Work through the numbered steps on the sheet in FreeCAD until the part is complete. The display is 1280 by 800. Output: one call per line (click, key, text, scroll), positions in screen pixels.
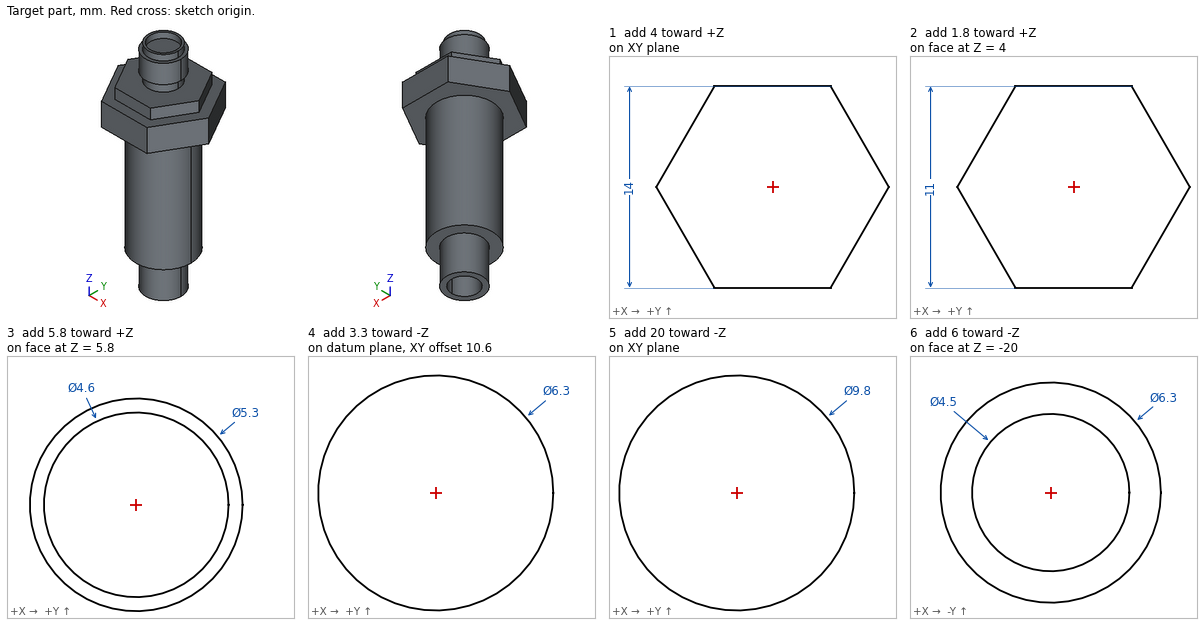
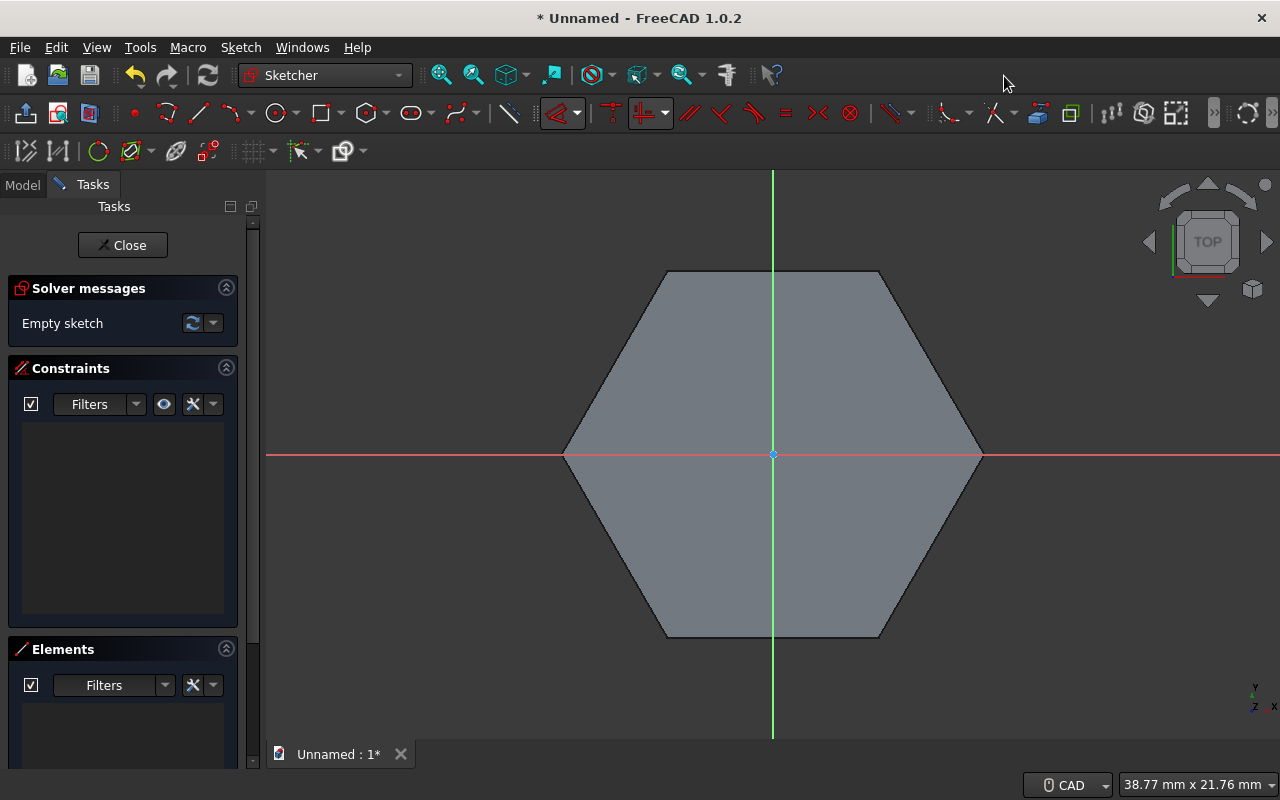
click(366, 114)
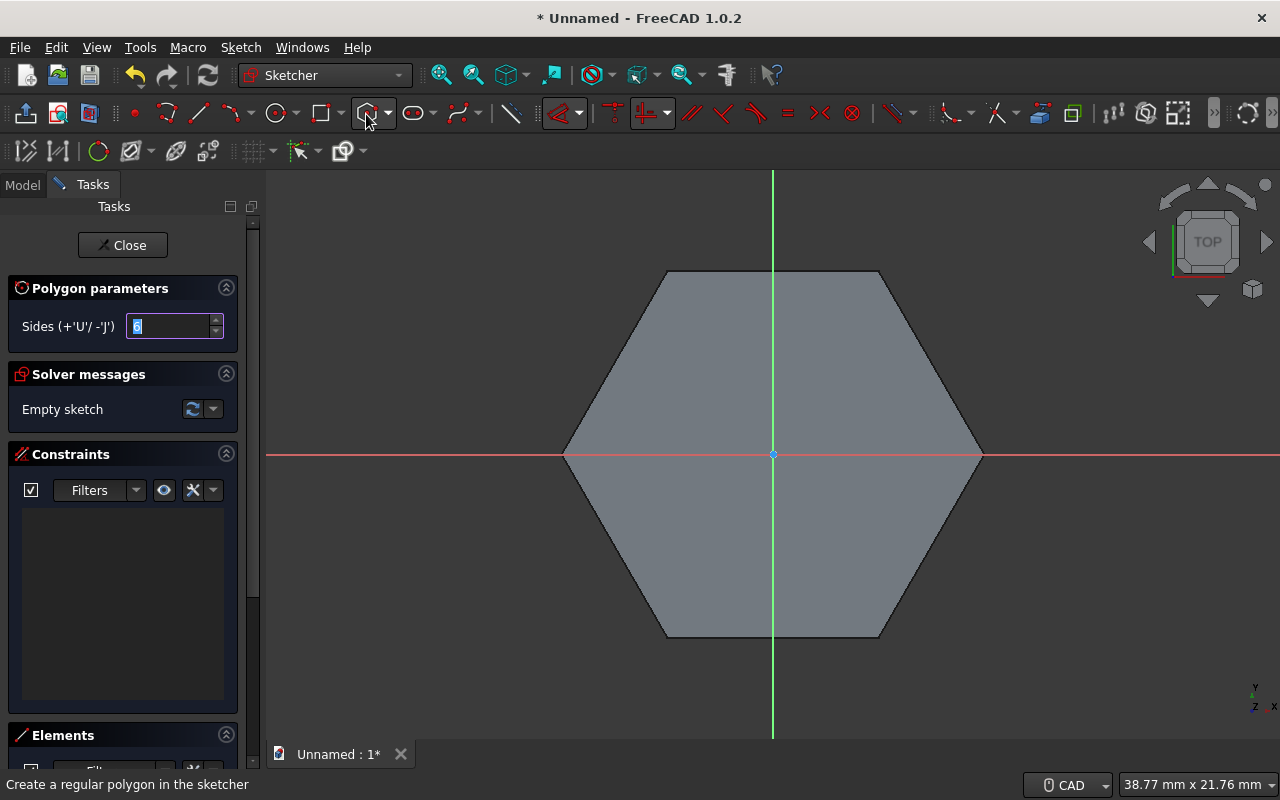
click(773, 454)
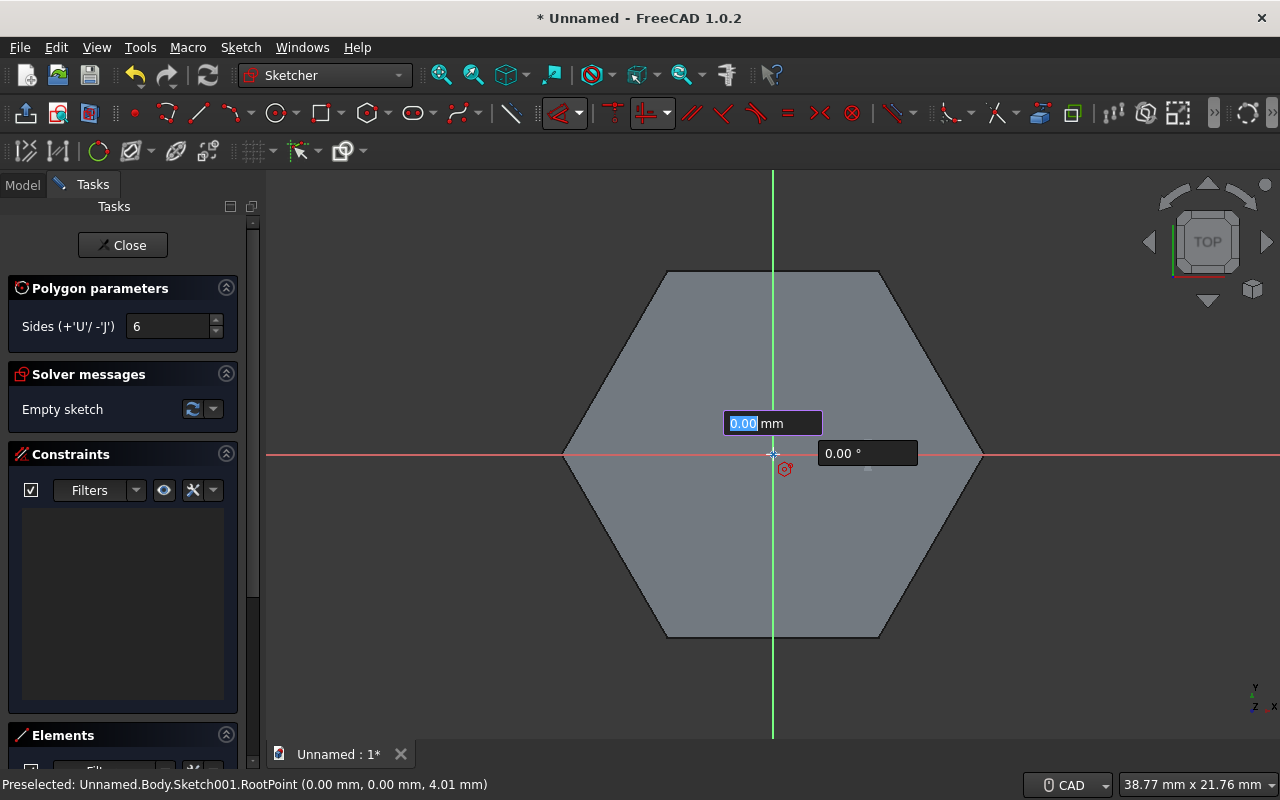
click(939, 454)
right_click(939, 454)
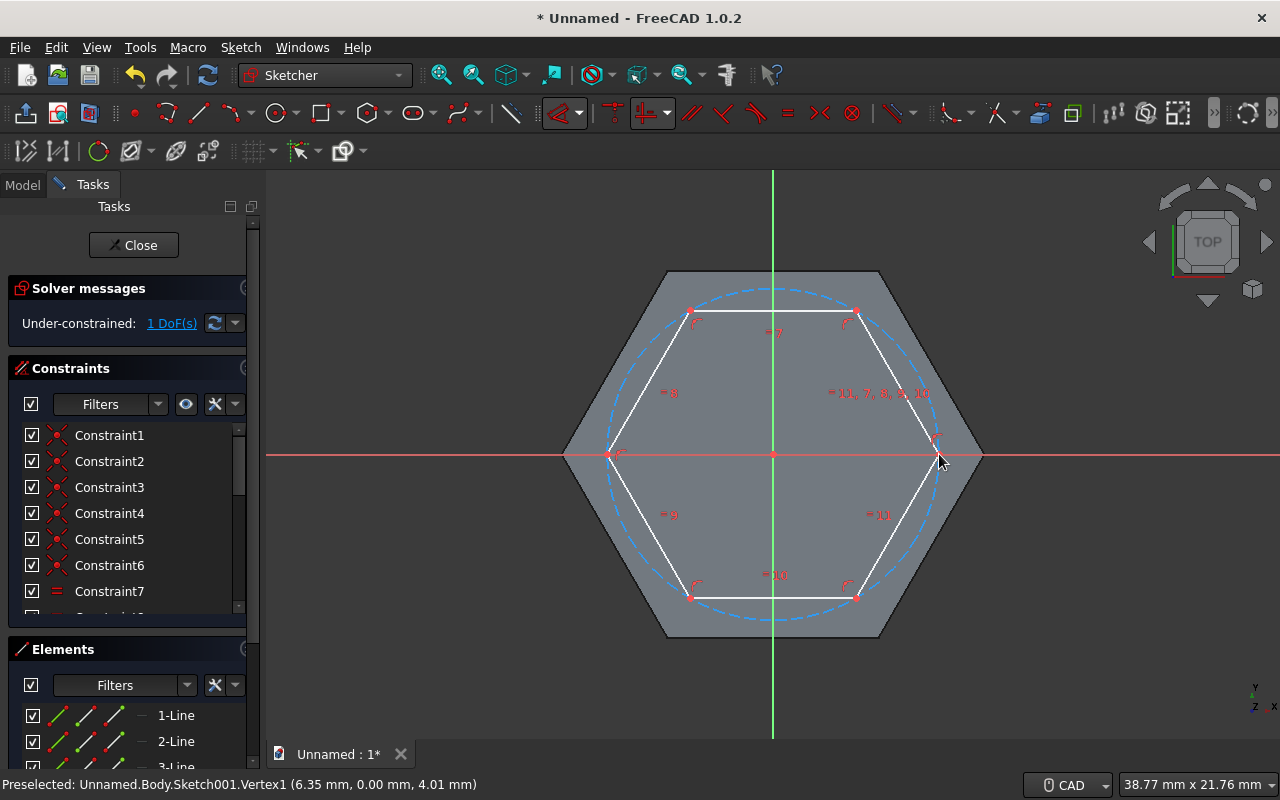
click(690, 598)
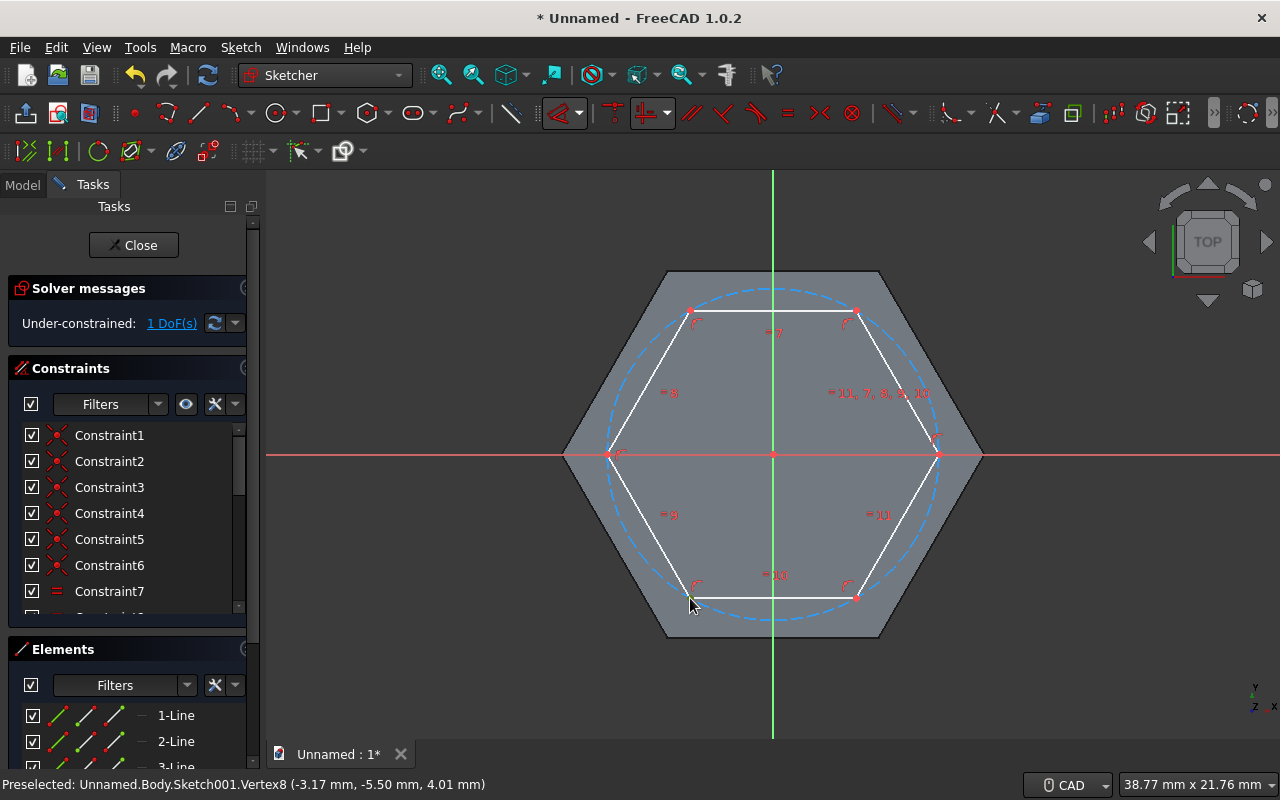
click(856, 311)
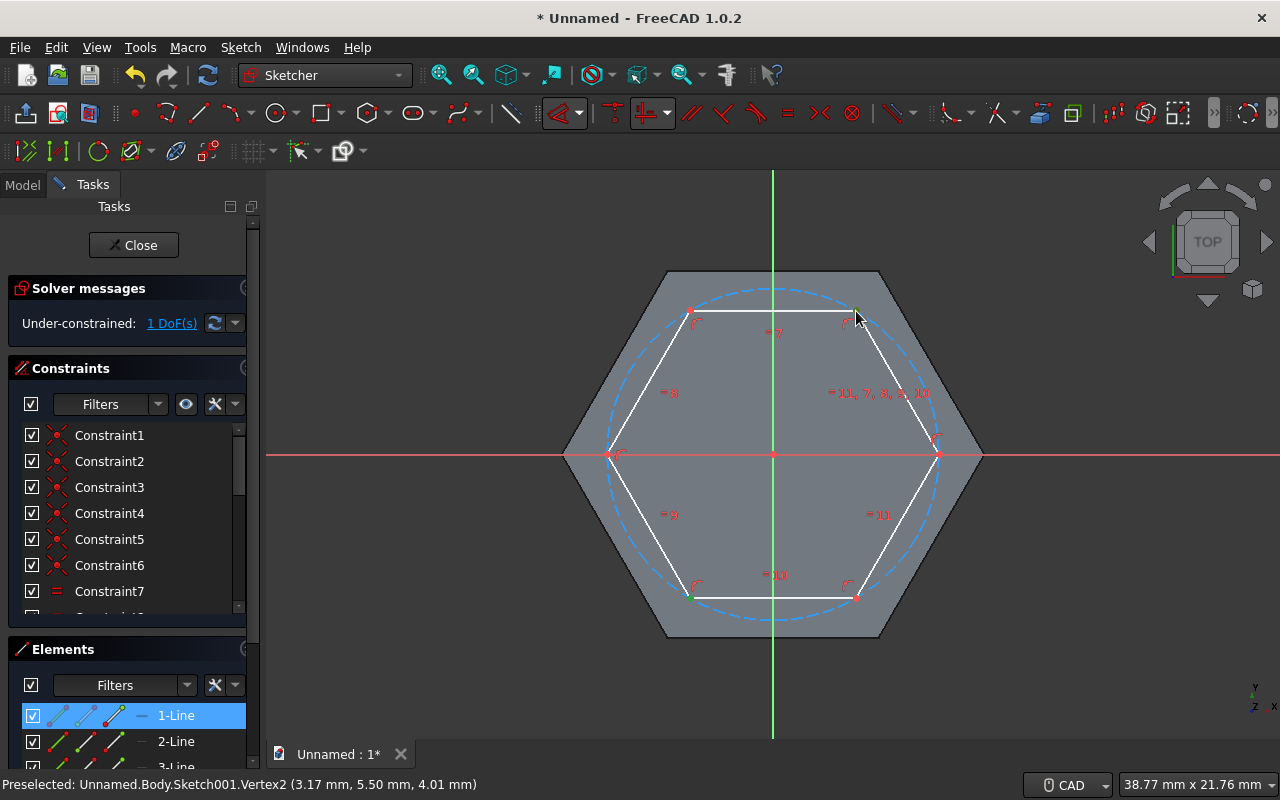
key(i)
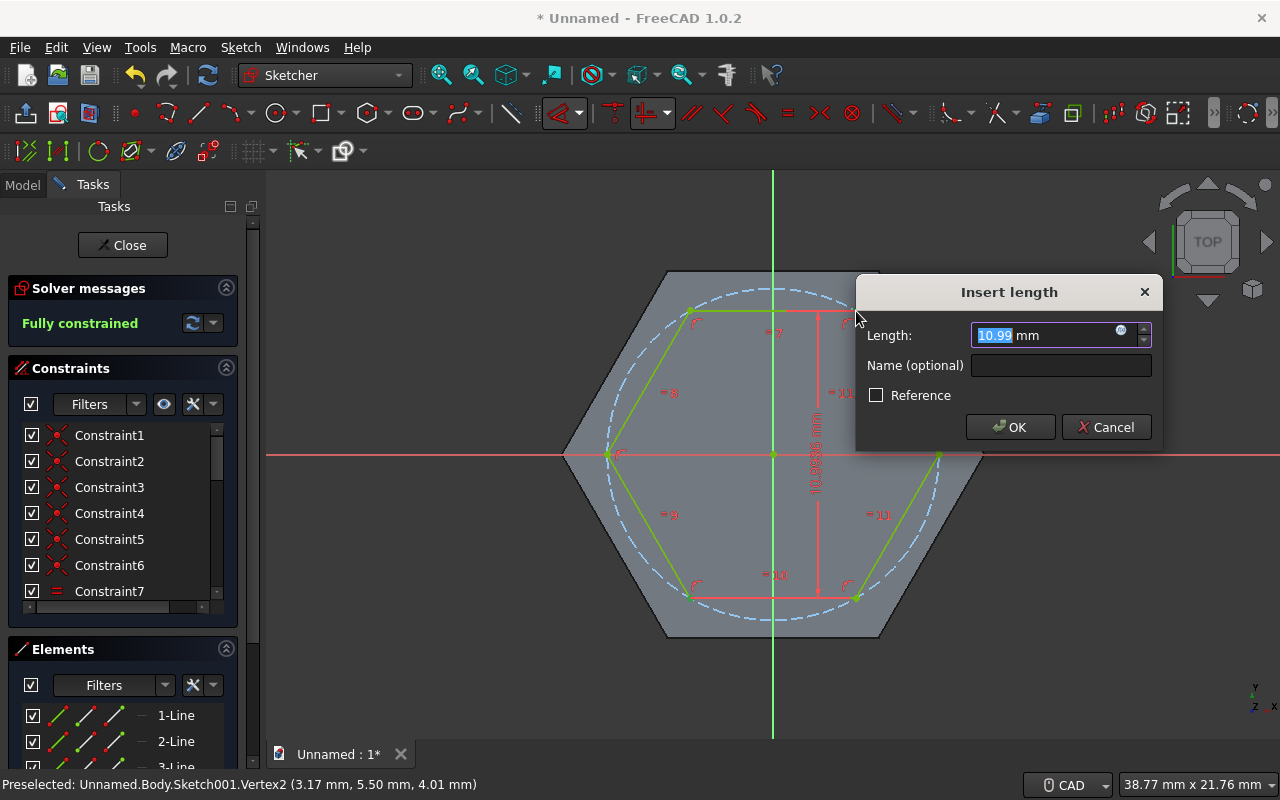
text(11)
key(Return)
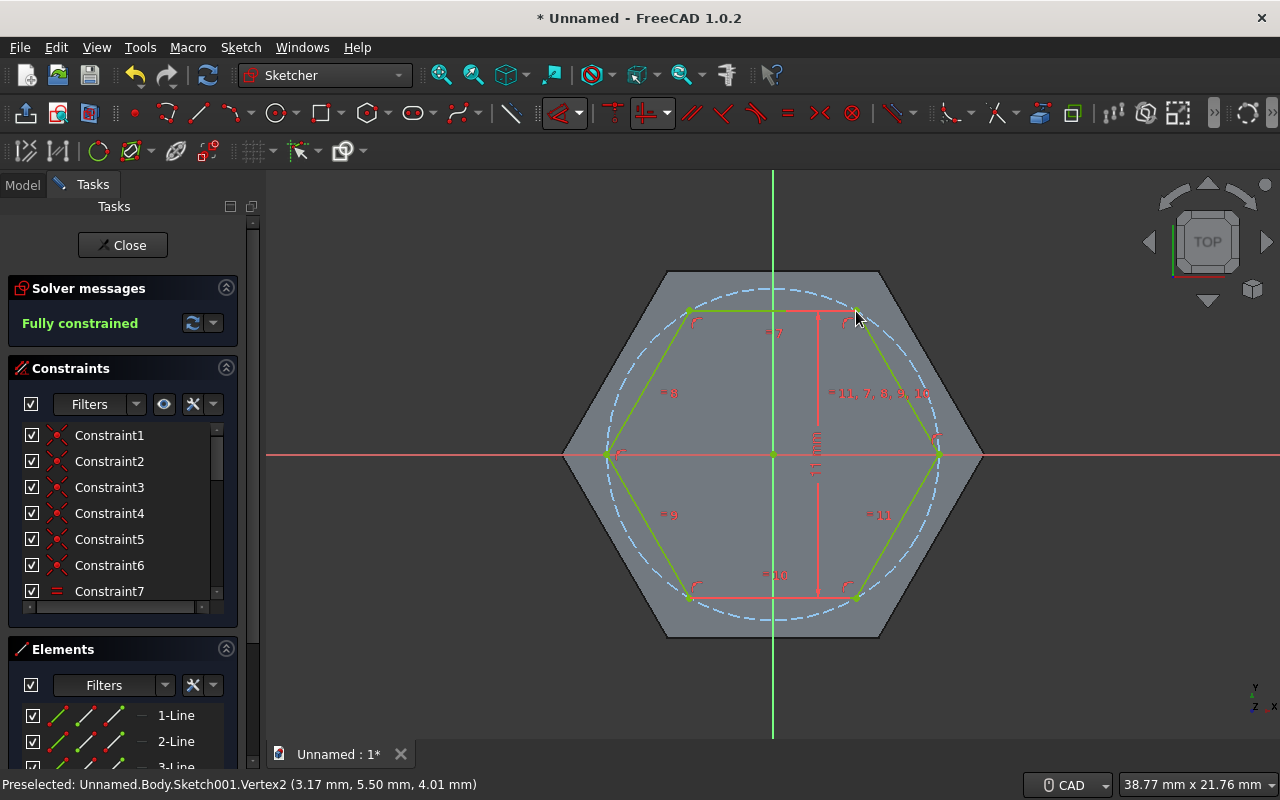
click(123, 245)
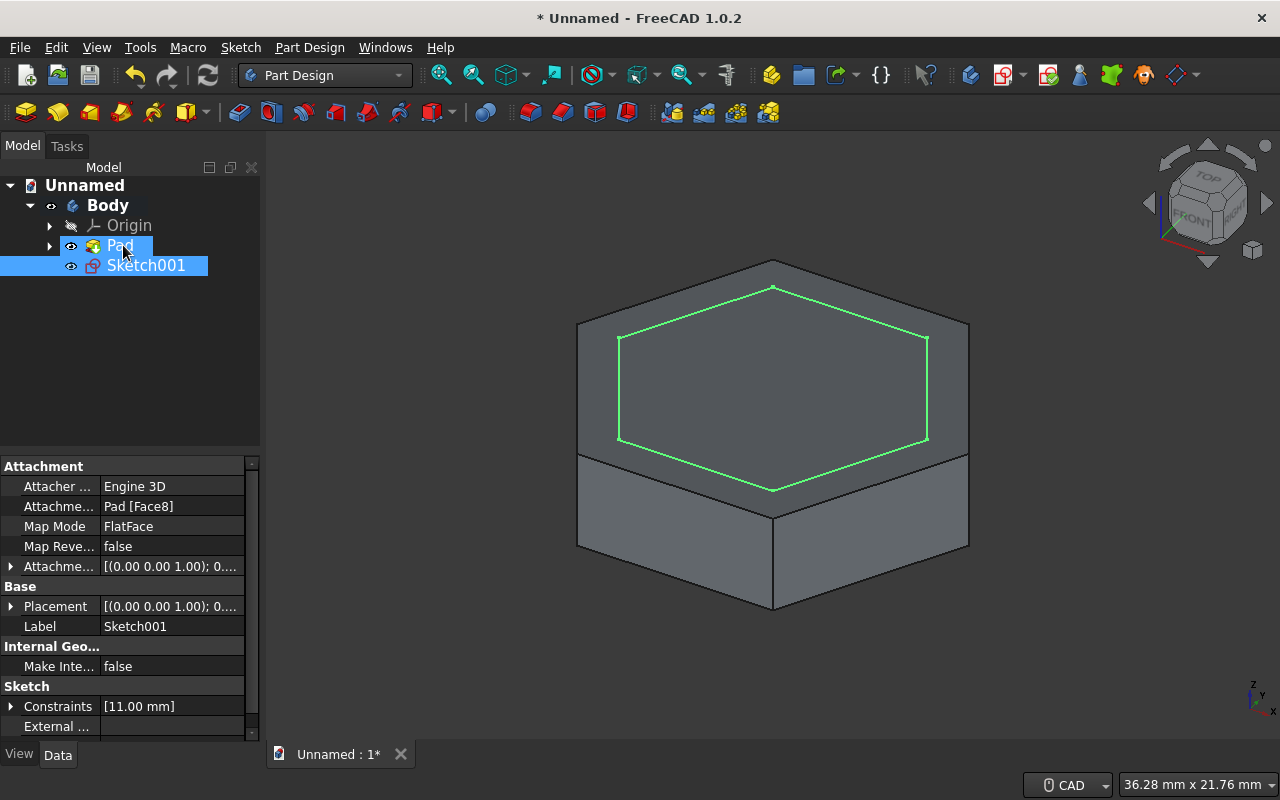
click(26, 112)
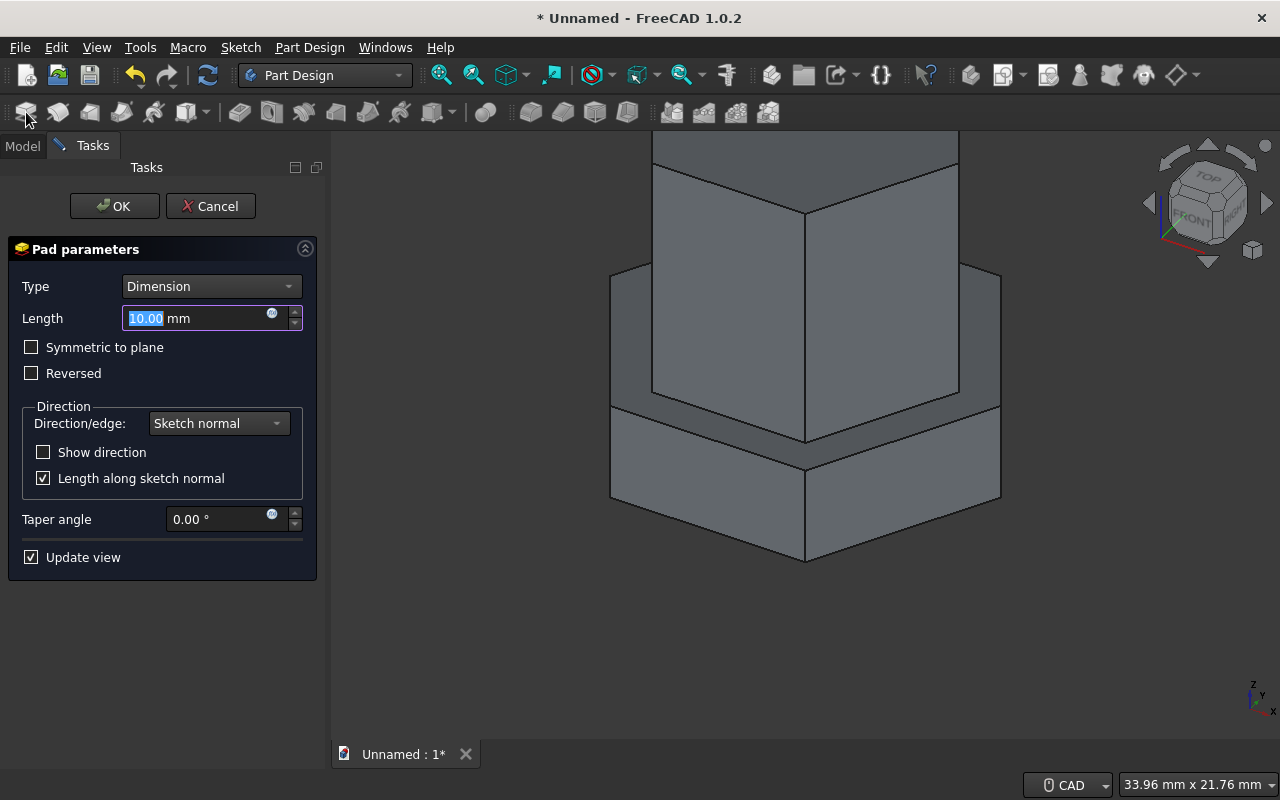
text(1.8)
key(Tab)